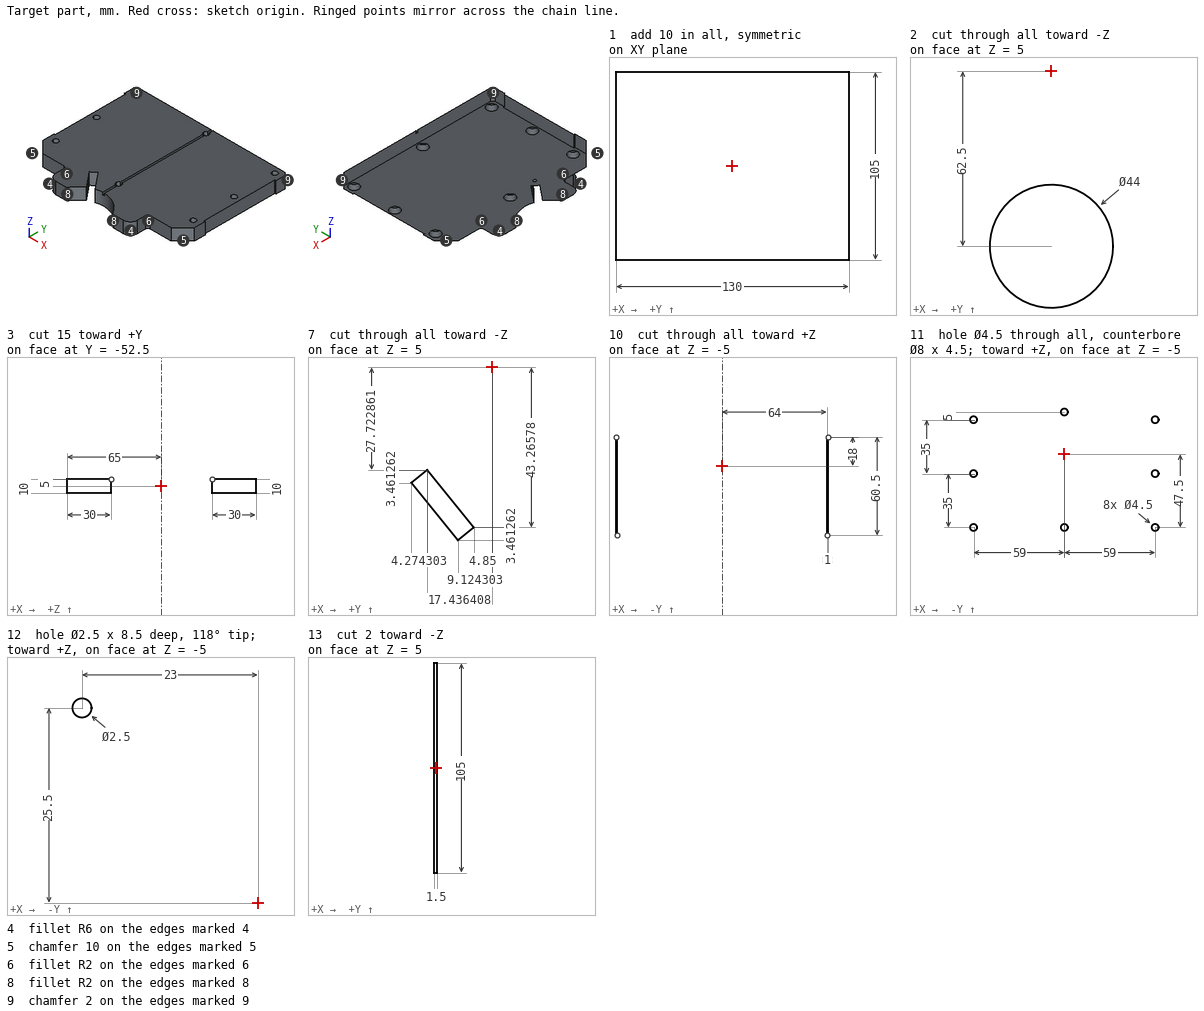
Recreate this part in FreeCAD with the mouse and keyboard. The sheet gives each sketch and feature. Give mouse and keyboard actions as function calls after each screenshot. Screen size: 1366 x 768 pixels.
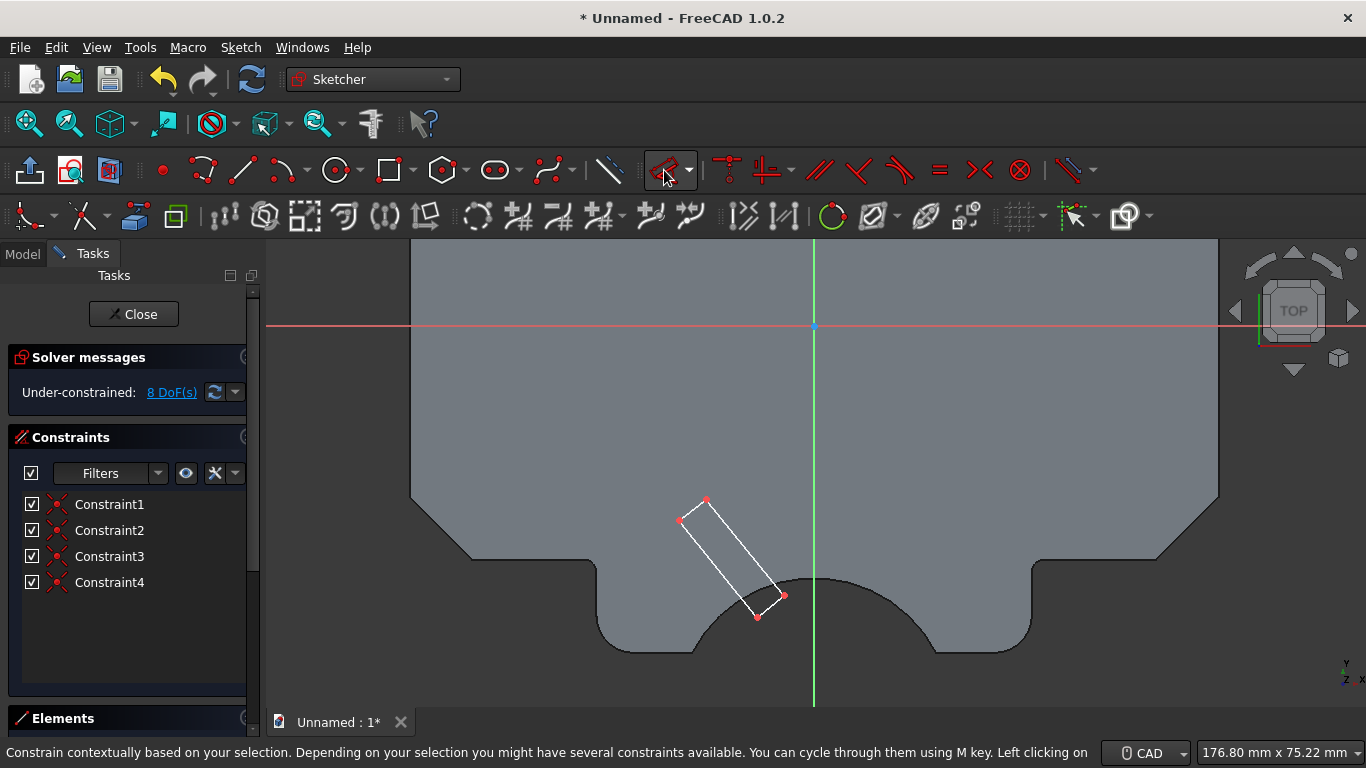
scroll(784, 596, up, 2)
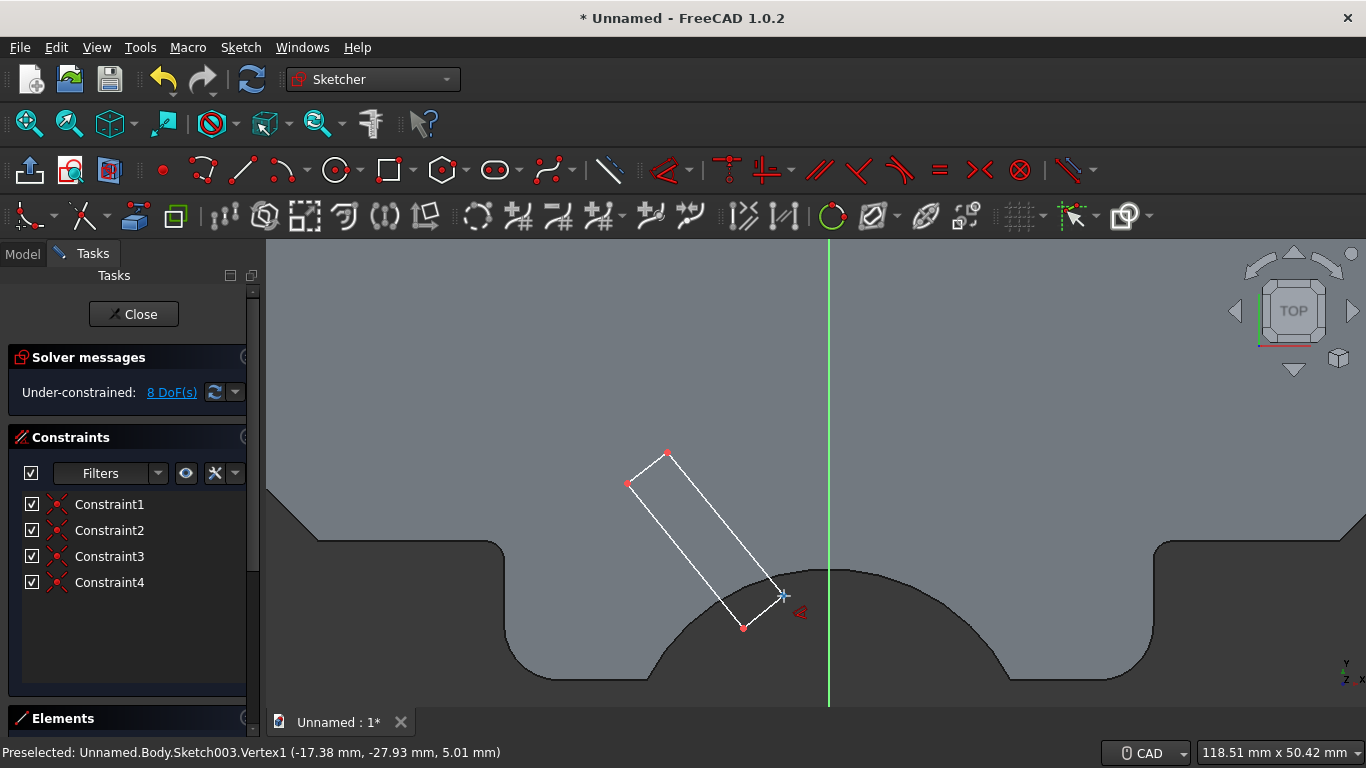
click(784, 596)
click(806, 630)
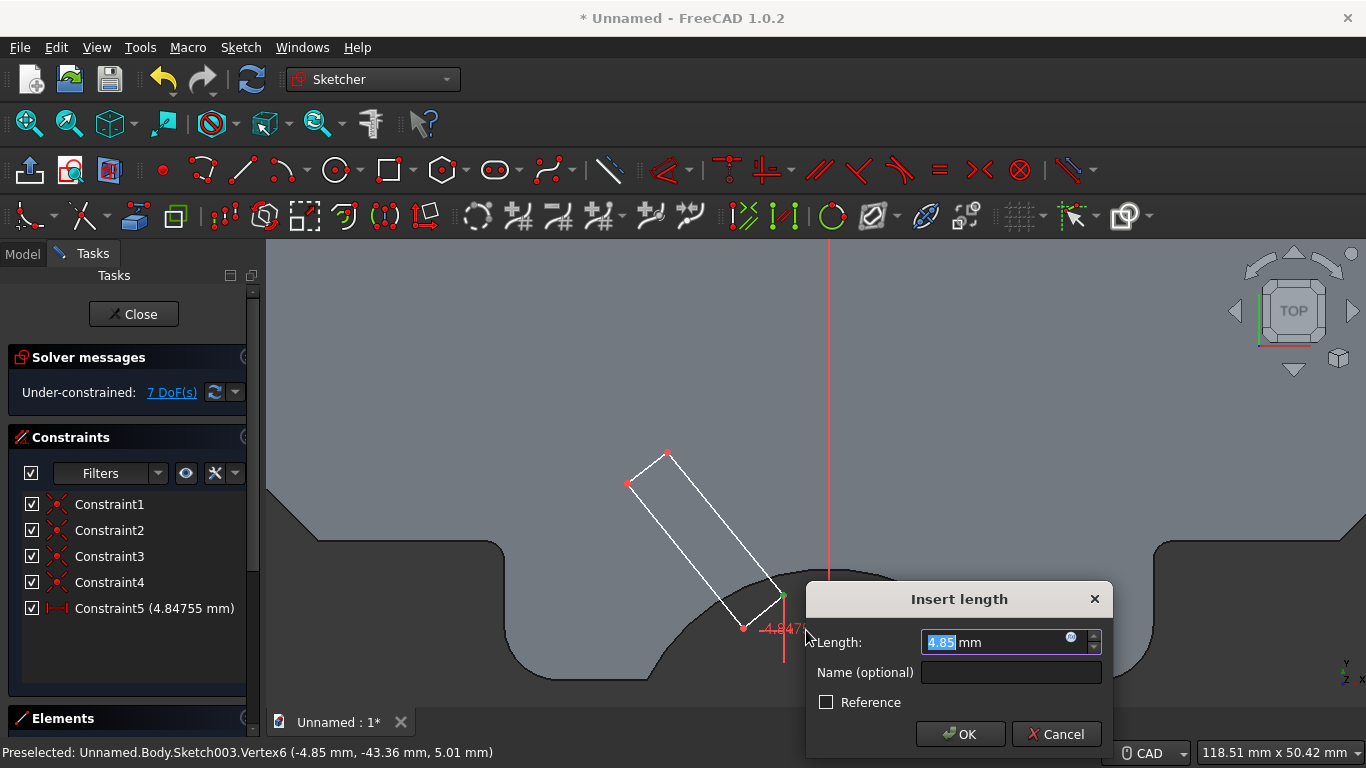
text(4.85)
key(Return)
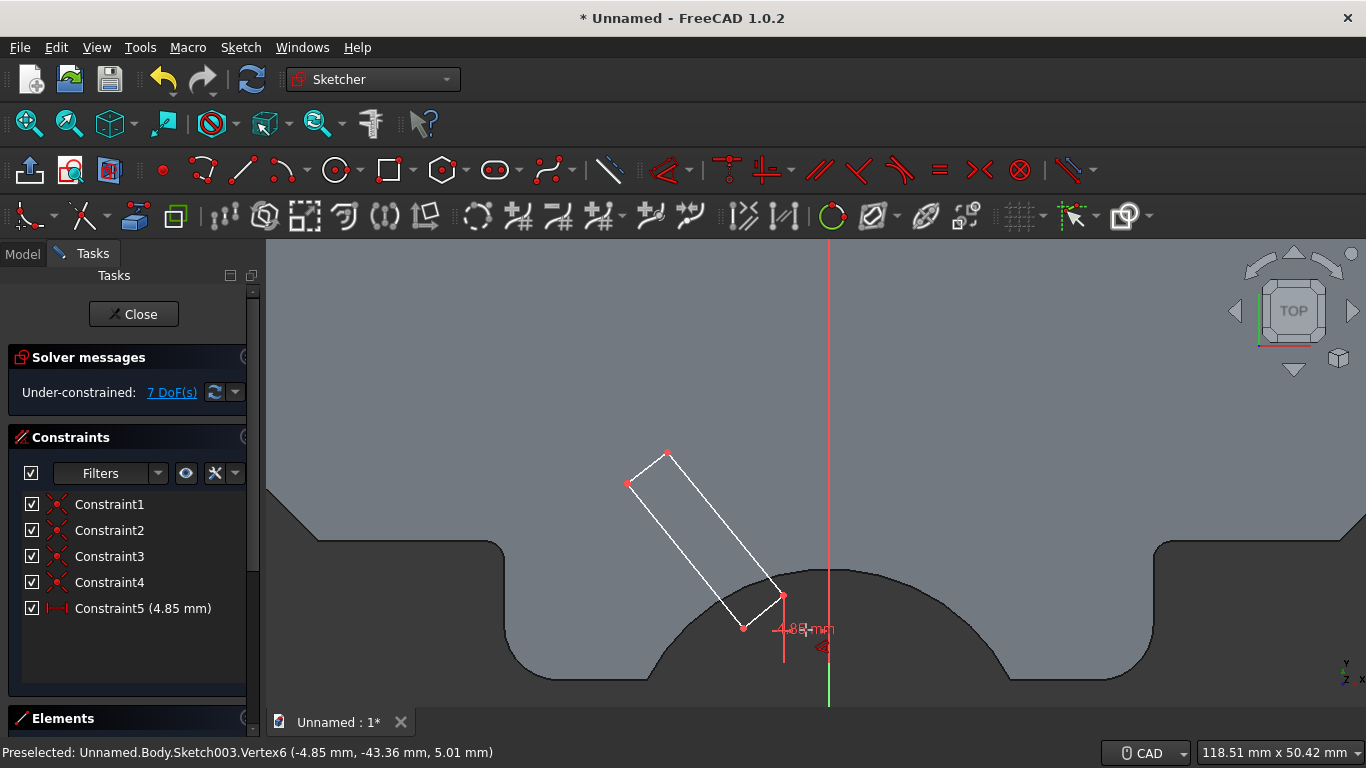
click(743, 628)
click(786, 662)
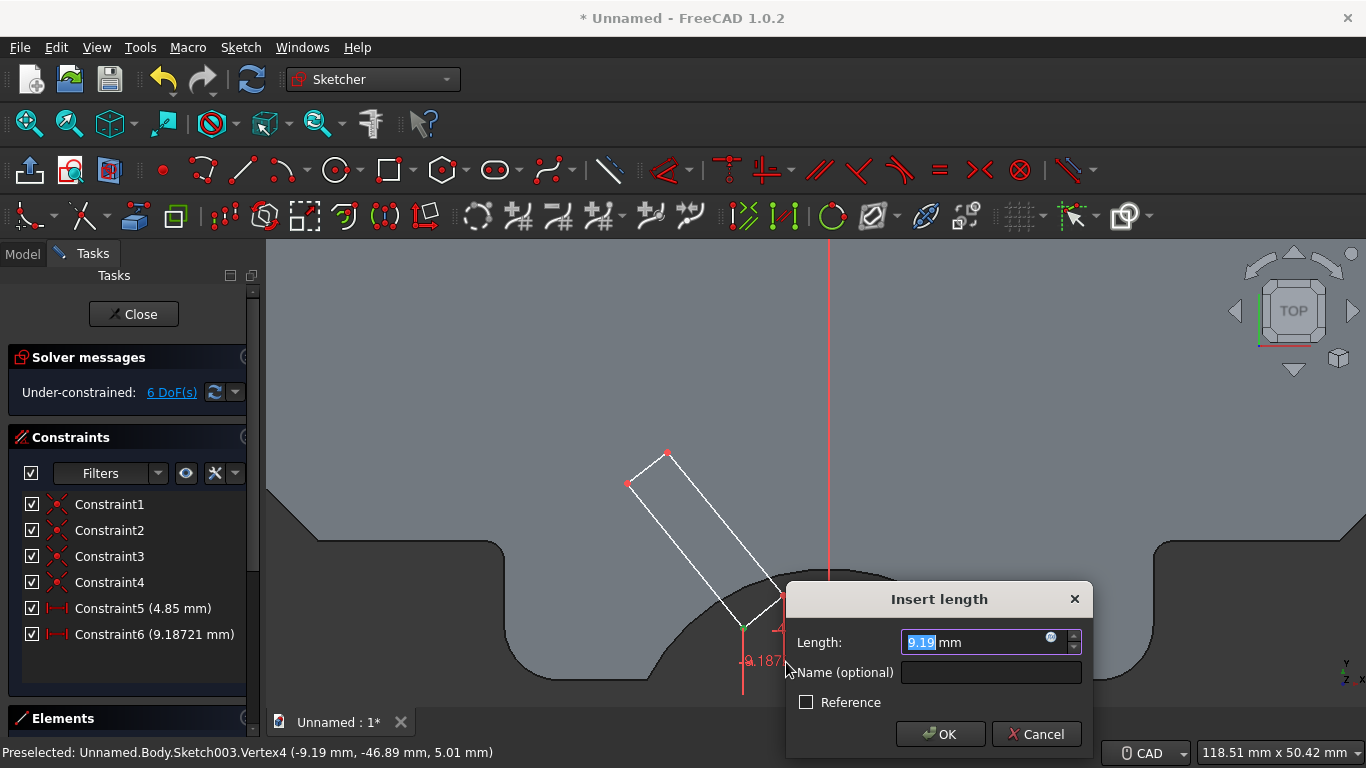
text(9.124303)
key(Return)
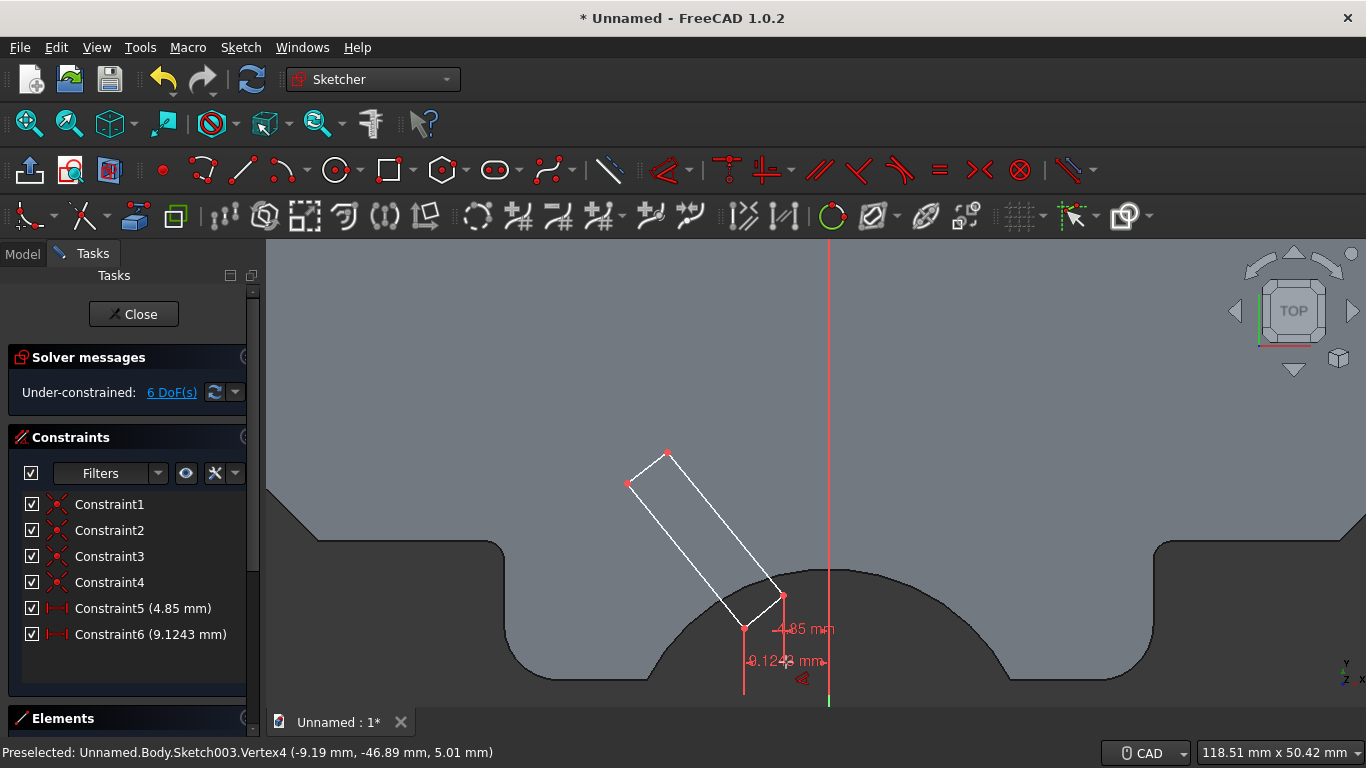
click(784, 596)
click(863, 431)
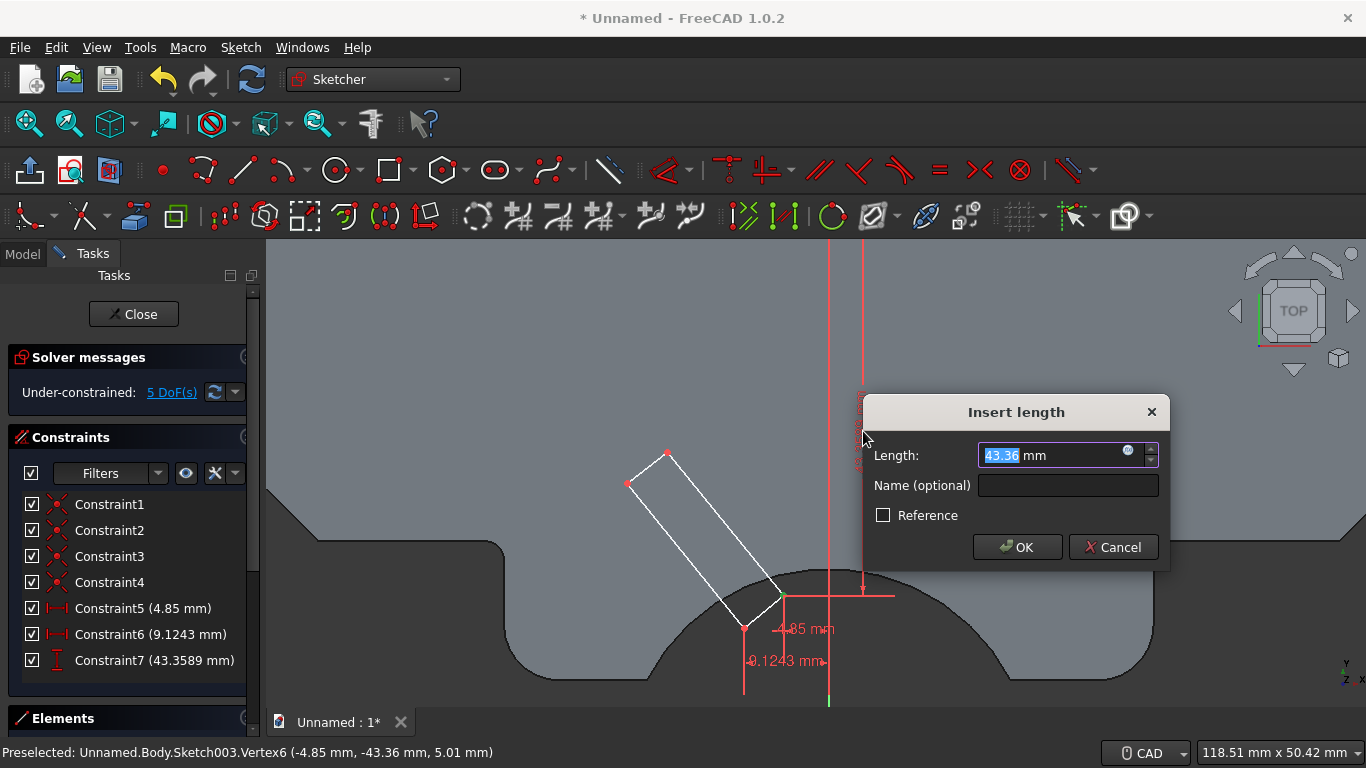
text(43.26578)
key(Return)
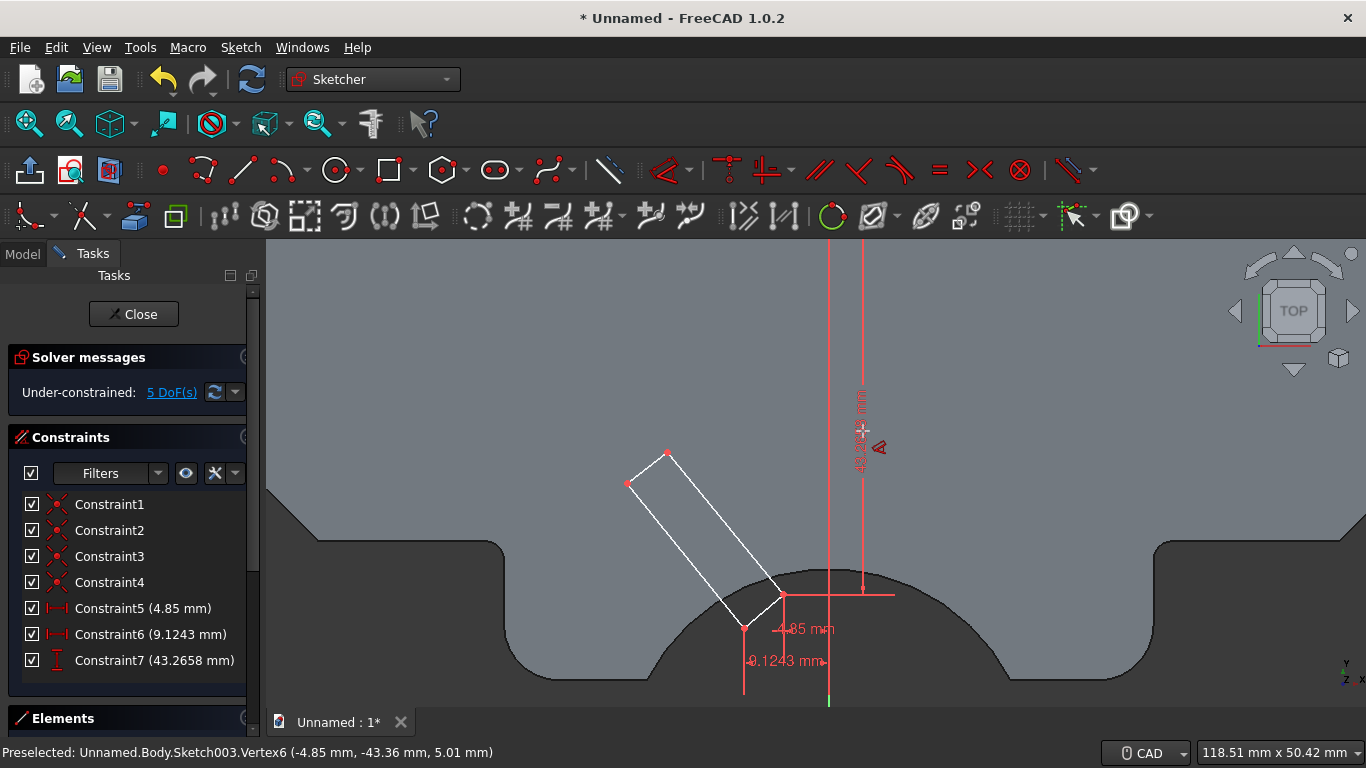
click(655, 462)
click(633, 518)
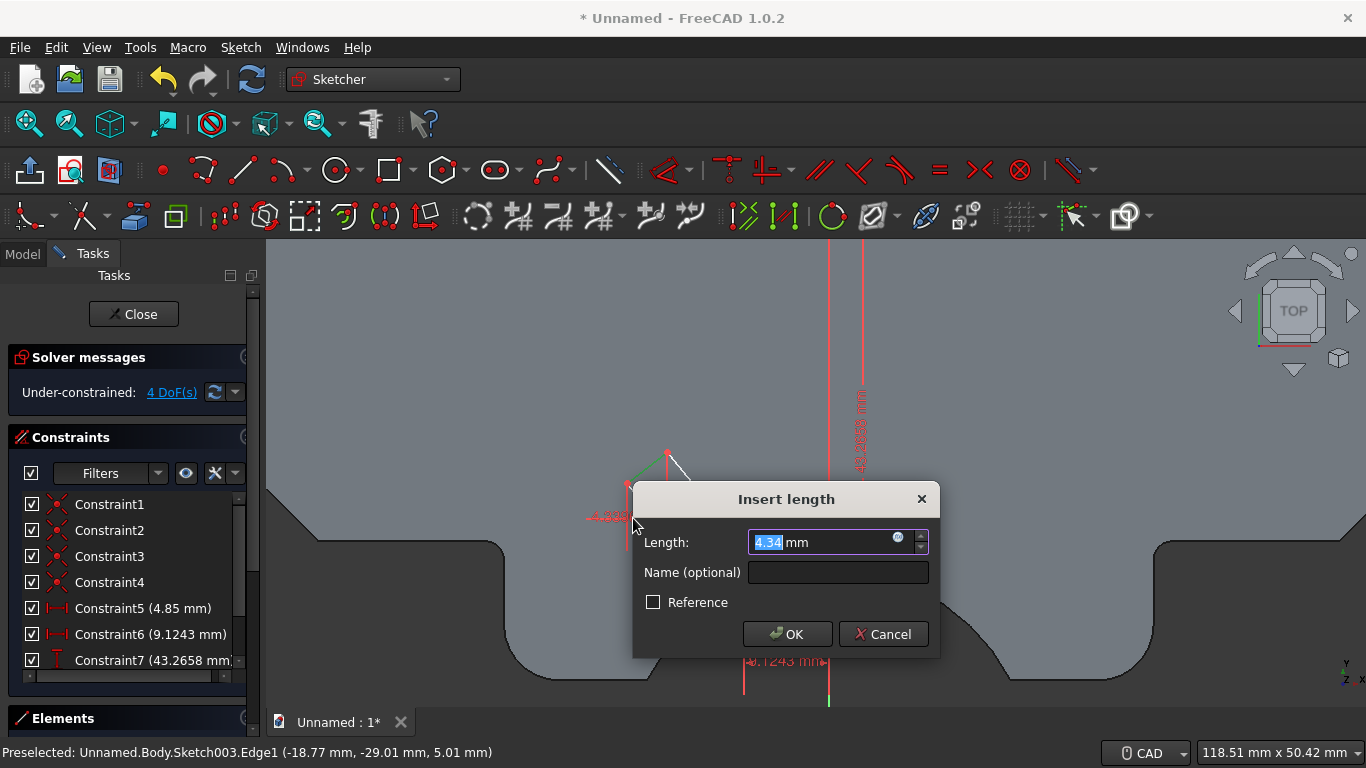
text(4.274303)
key(Return)